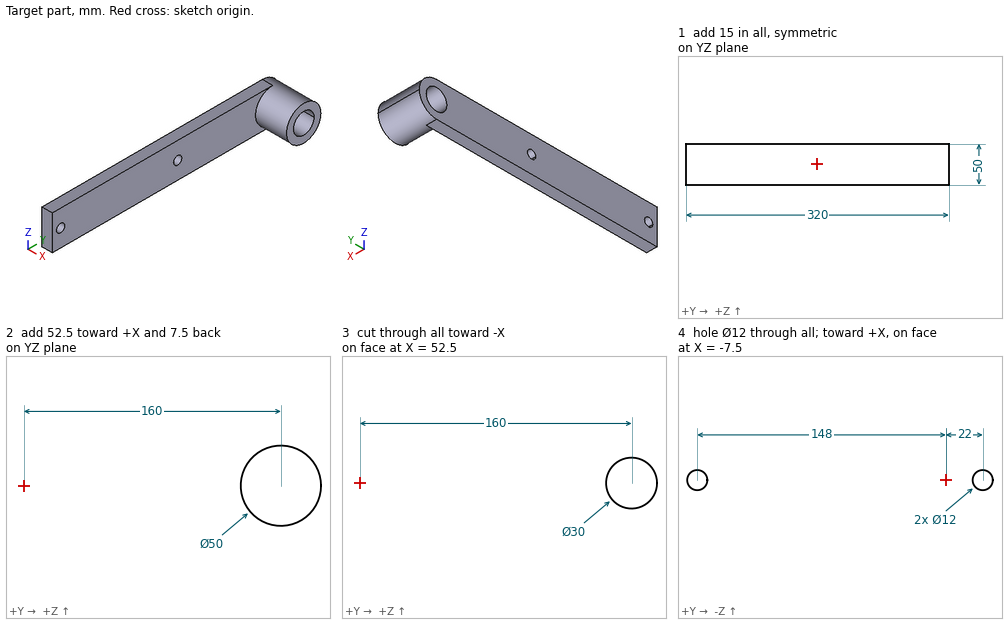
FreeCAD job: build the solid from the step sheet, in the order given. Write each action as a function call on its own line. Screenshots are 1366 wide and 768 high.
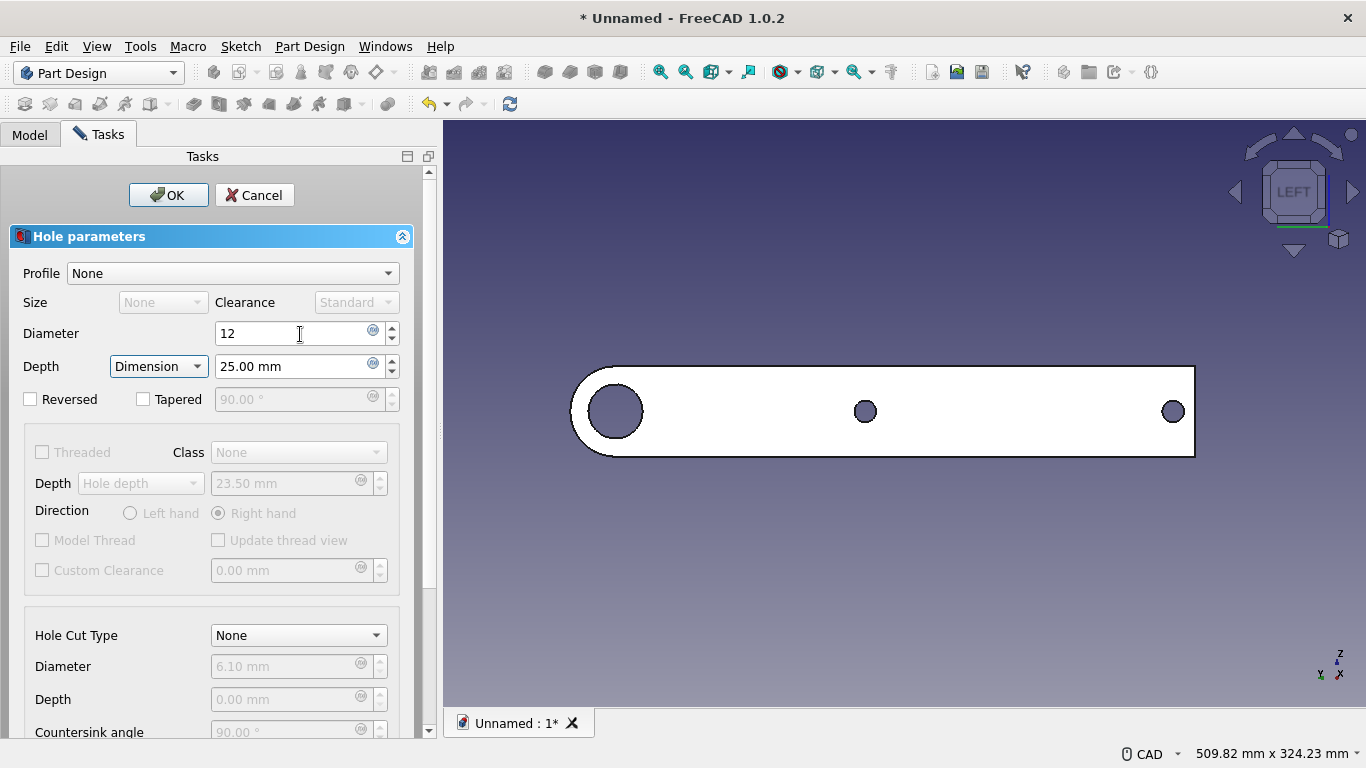
click(160, 366)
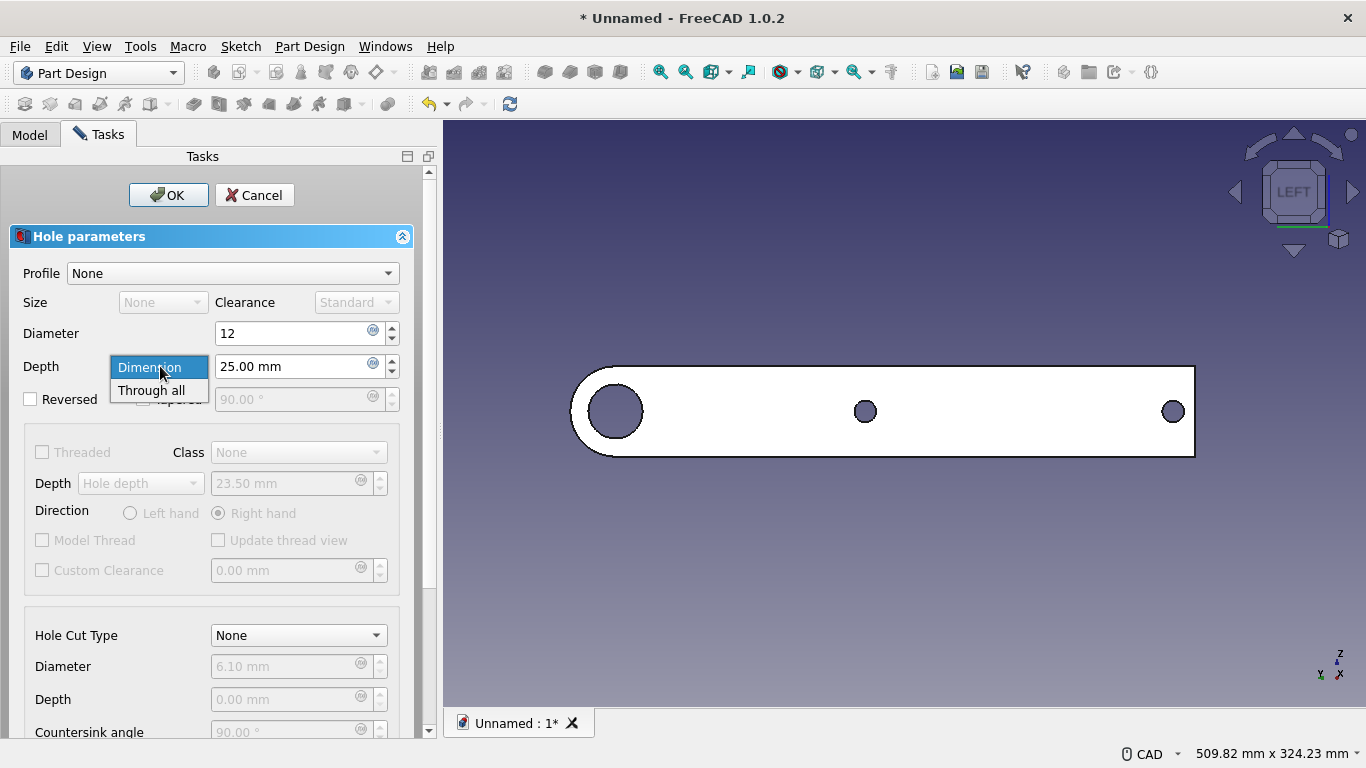
click(158, 390)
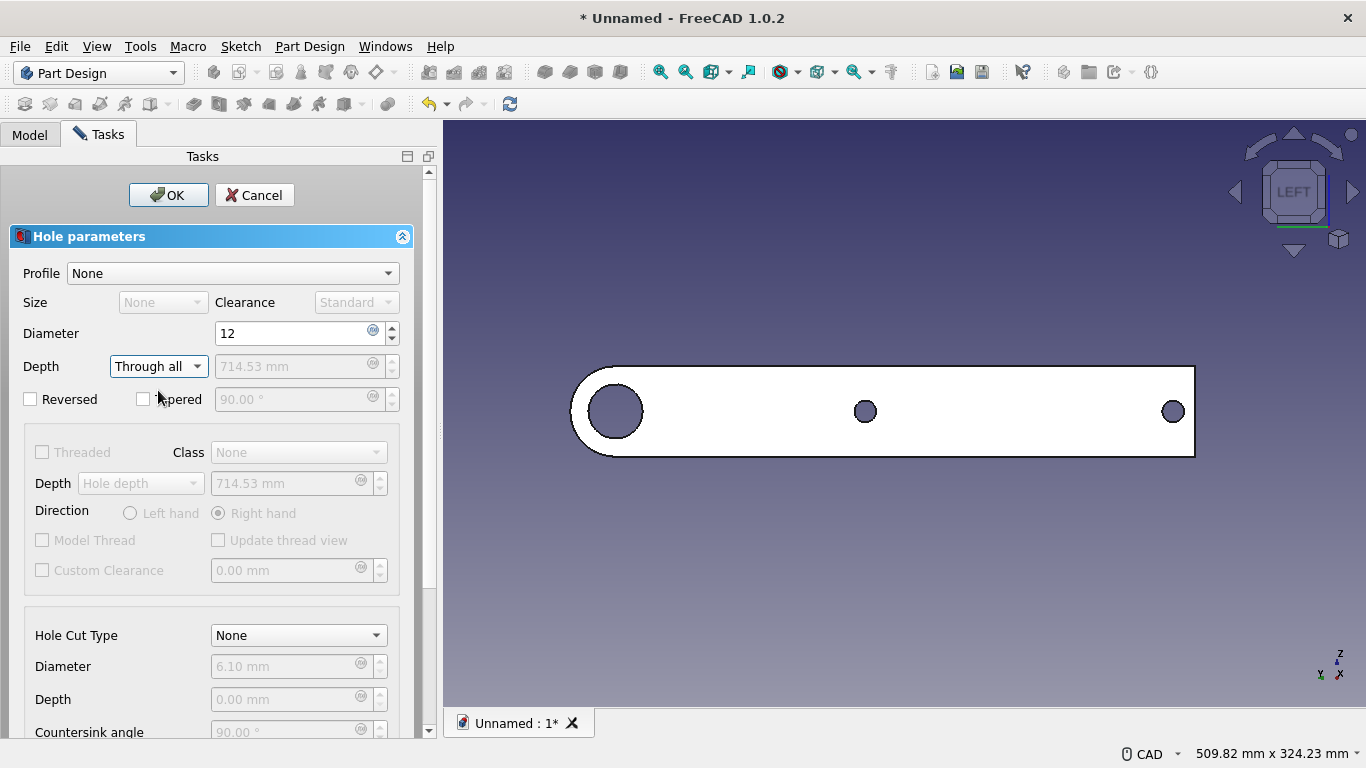
click(169, 195)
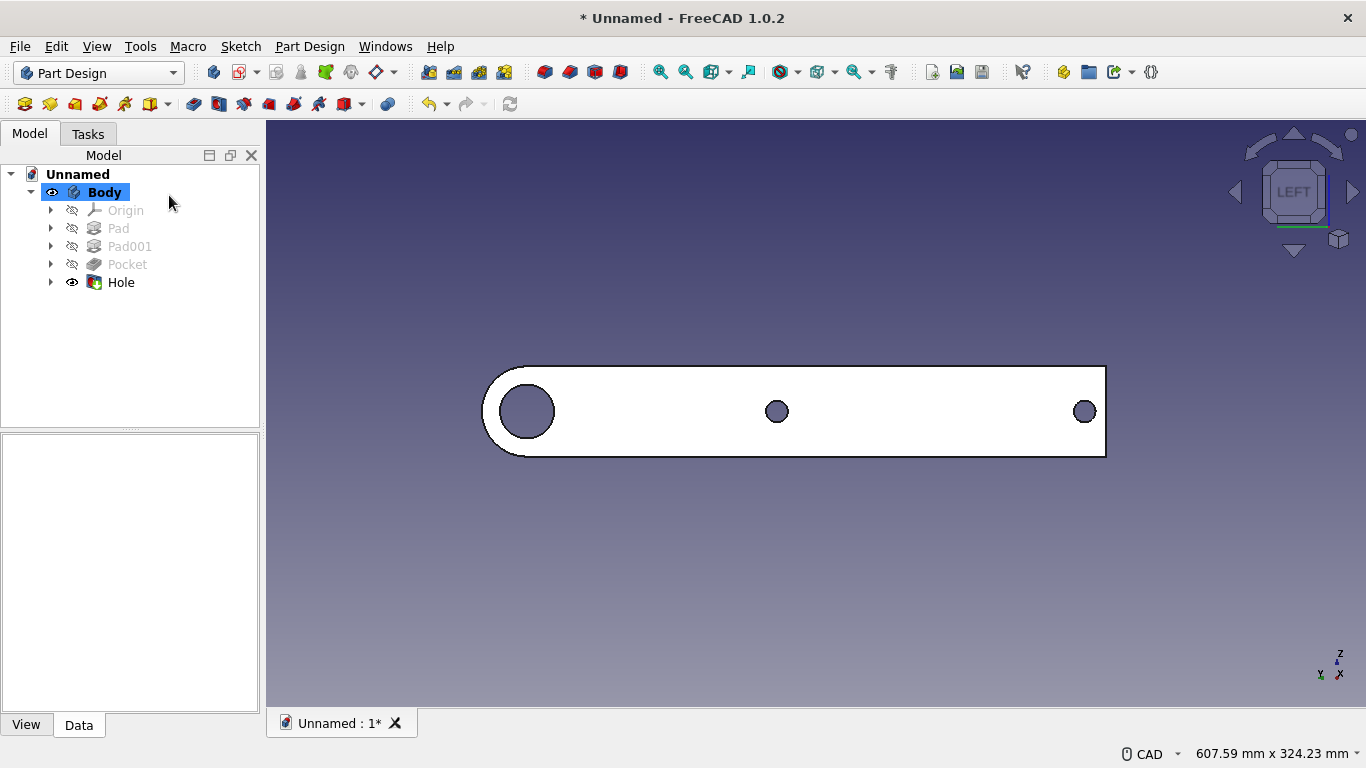
key(0)